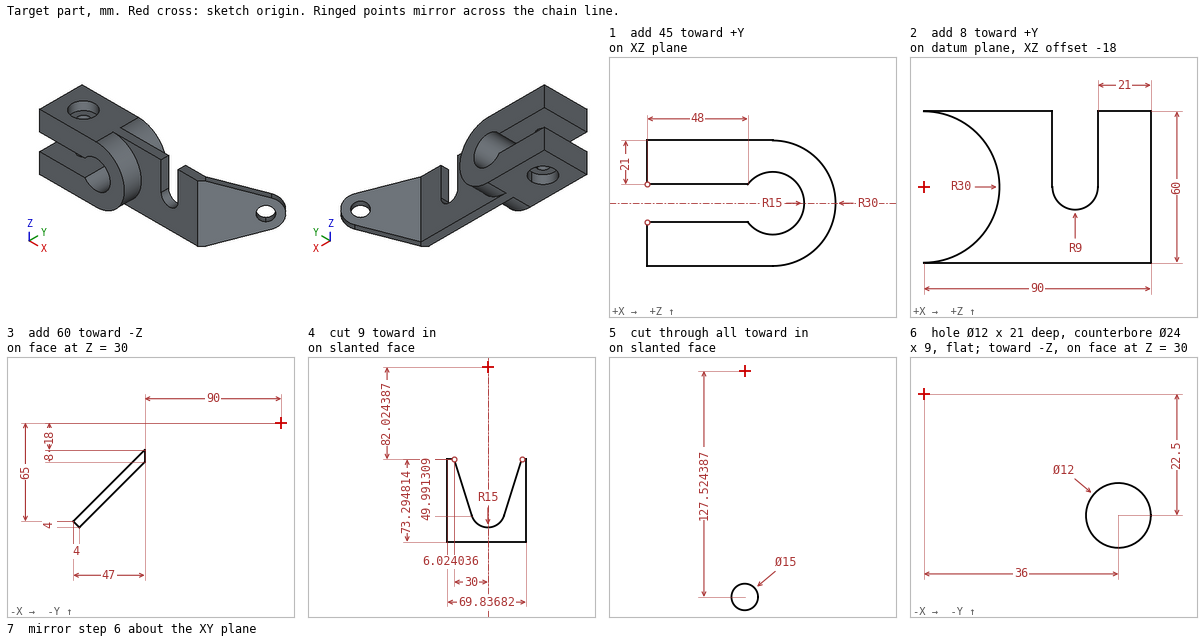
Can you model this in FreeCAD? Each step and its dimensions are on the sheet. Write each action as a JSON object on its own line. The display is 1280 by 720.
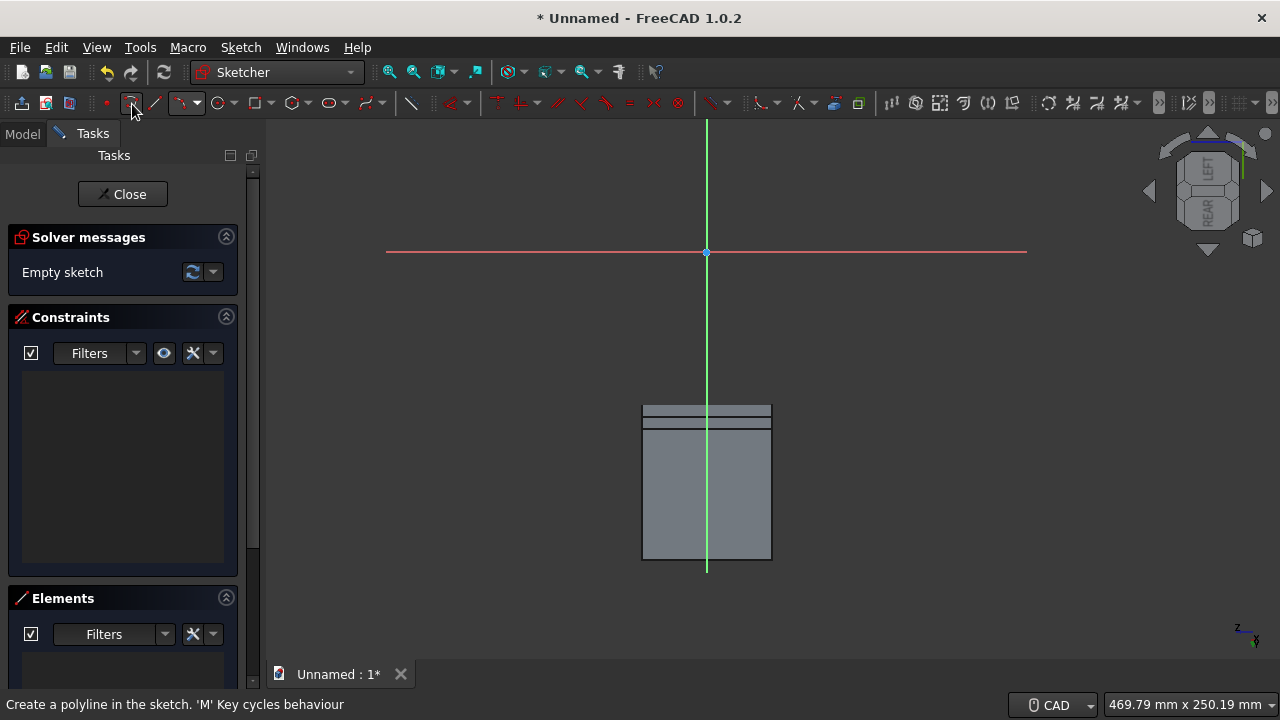
{"action": "left_click", "coordinate": [676, 537]}
{"action": "left_click", "coordinate": [642, 429]}
{"action": "left_click", "coordinate": [629, 429]}
{"action": "left_click", "coordinate": [629, 587]}
{"action": "left_click", "coordinate": [780, 587]}
{"action": "left_click", "coordinate": [780, 429]}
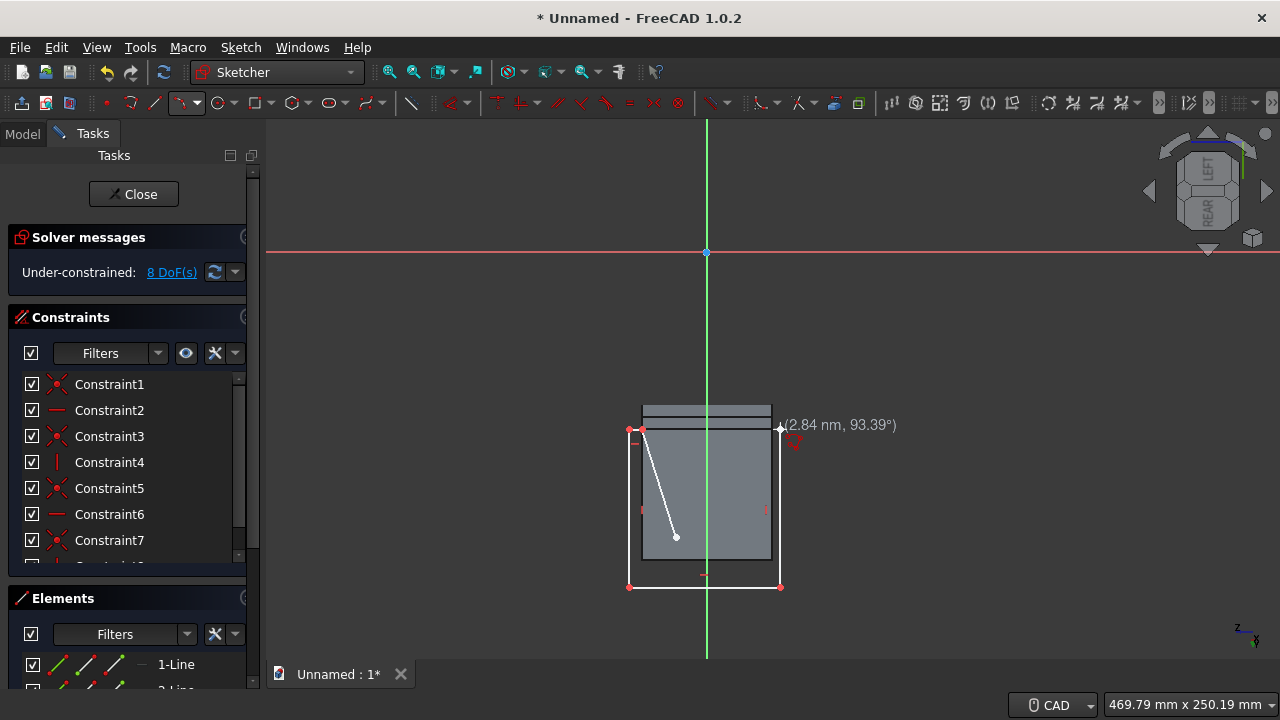
{"action": "scroll", "coordinate": [772, 429], "scroll_direction": "up", "scroll_amount": 4}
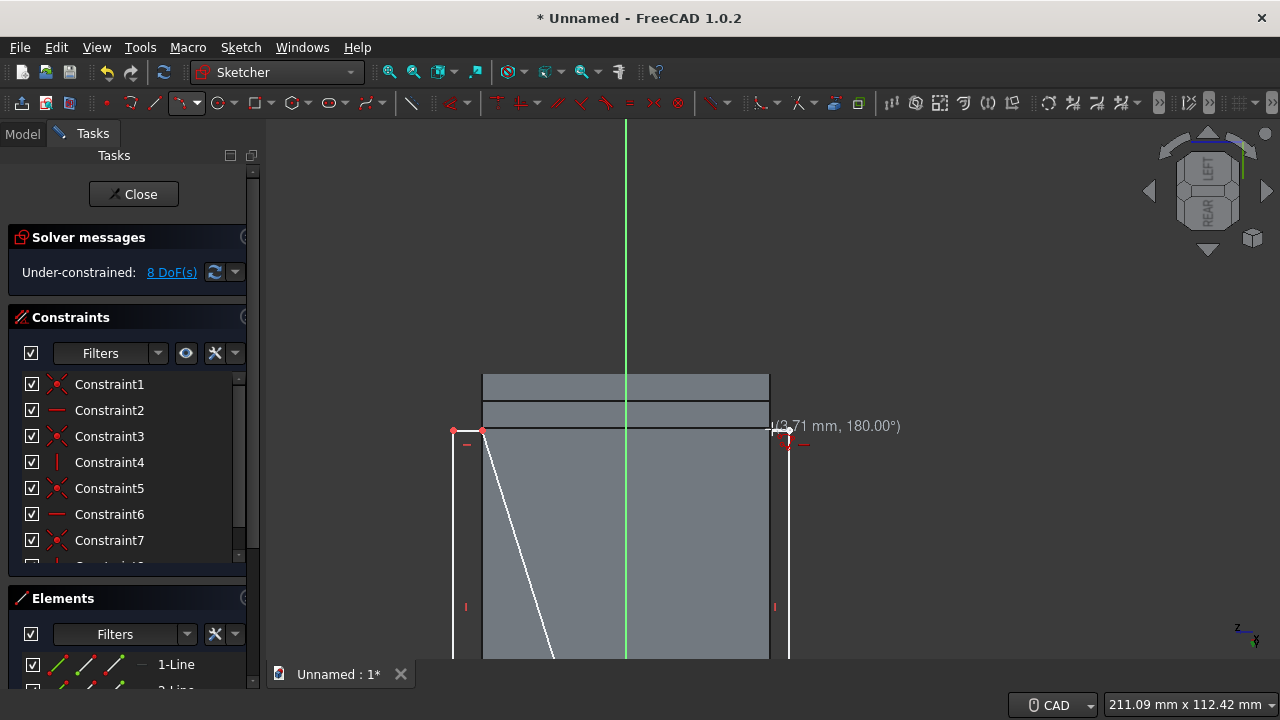
{"action": "left_click", "coordinate": [770, 428]}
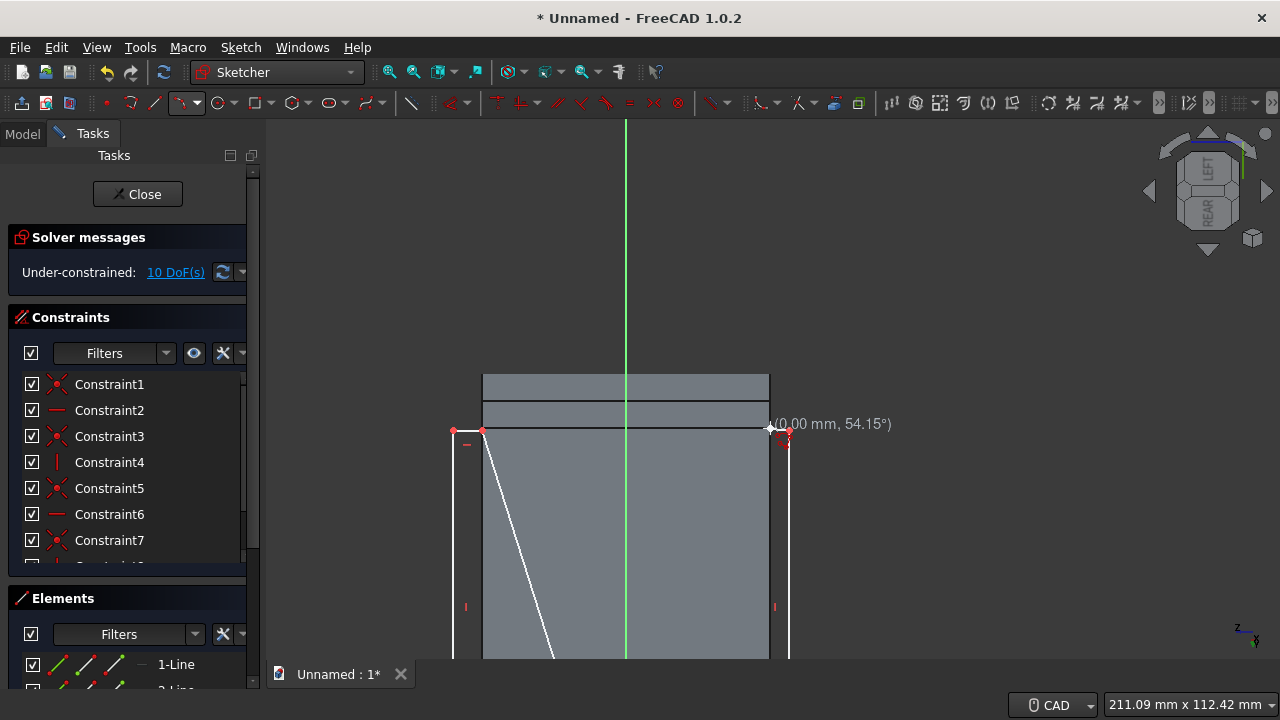
{"action": "scroll", "coordinate": [773, 374], "scroll_direction": "down", "scroll_amount": 4}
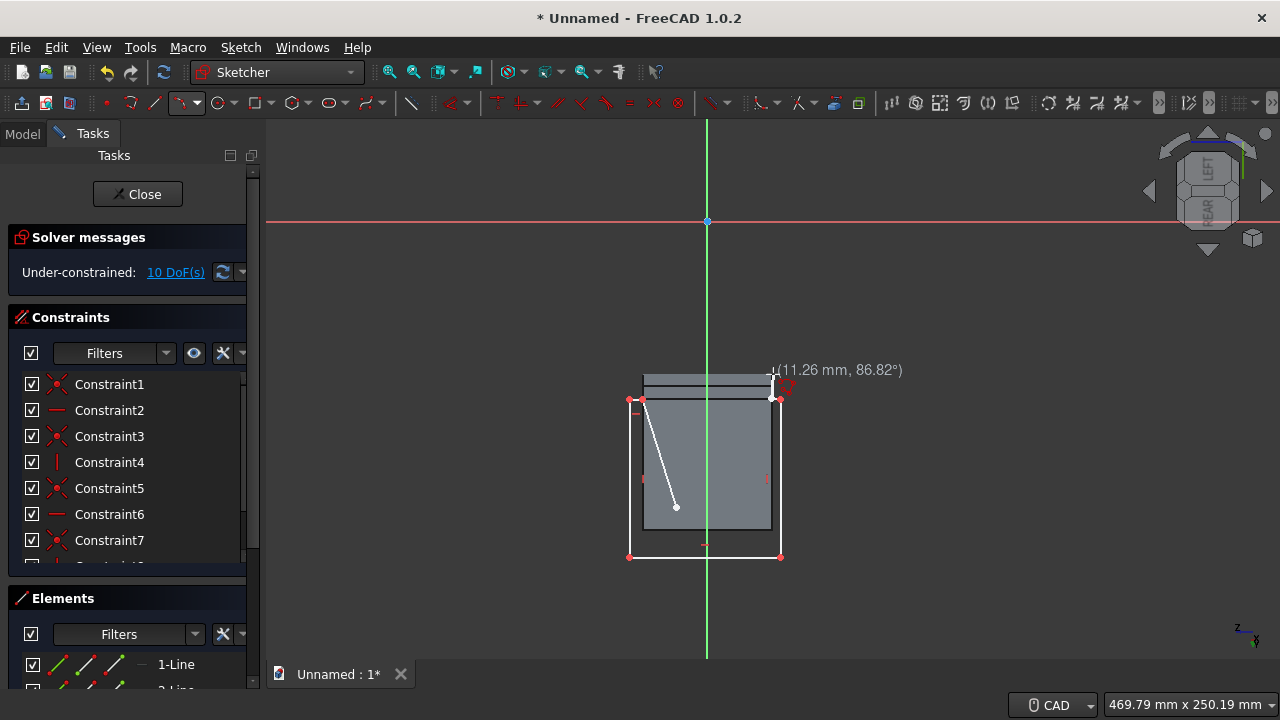
{"action": "left_click", "coordinate": [738, 507]}
{"action": "right_click", "coordinate": [738, 507]}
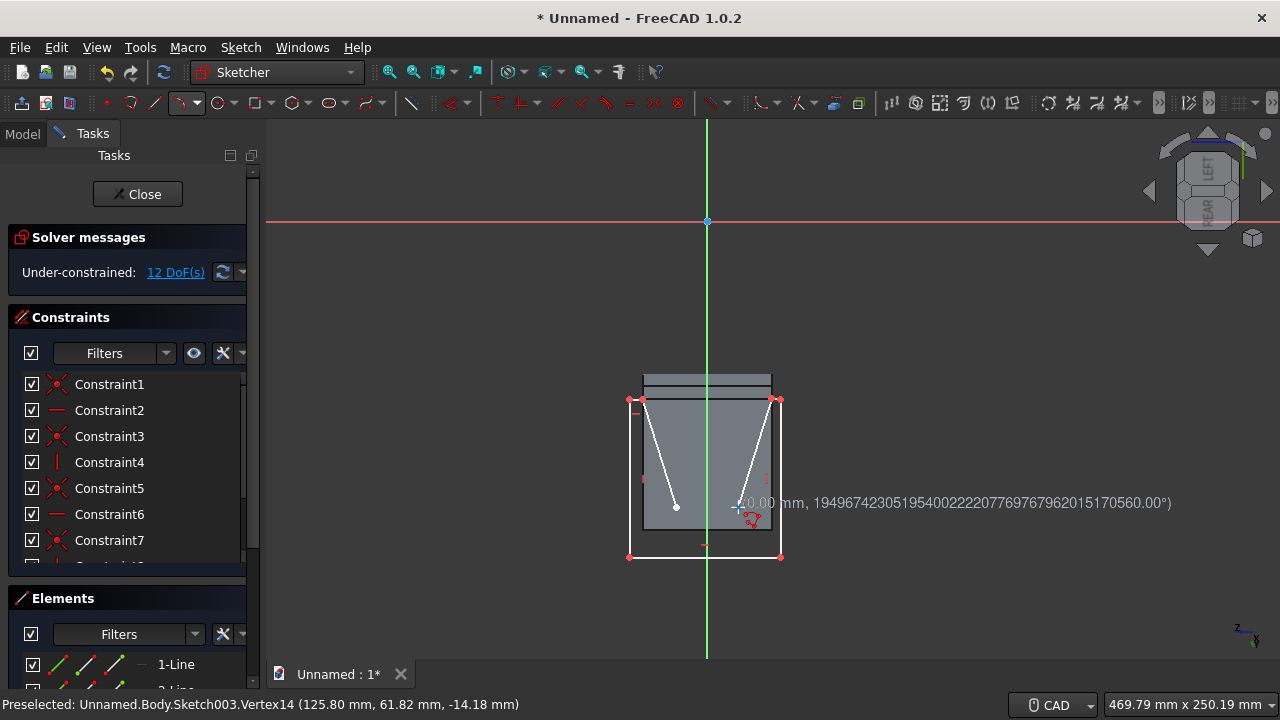
{"action": "left_click", "coordinate": [180, 104]}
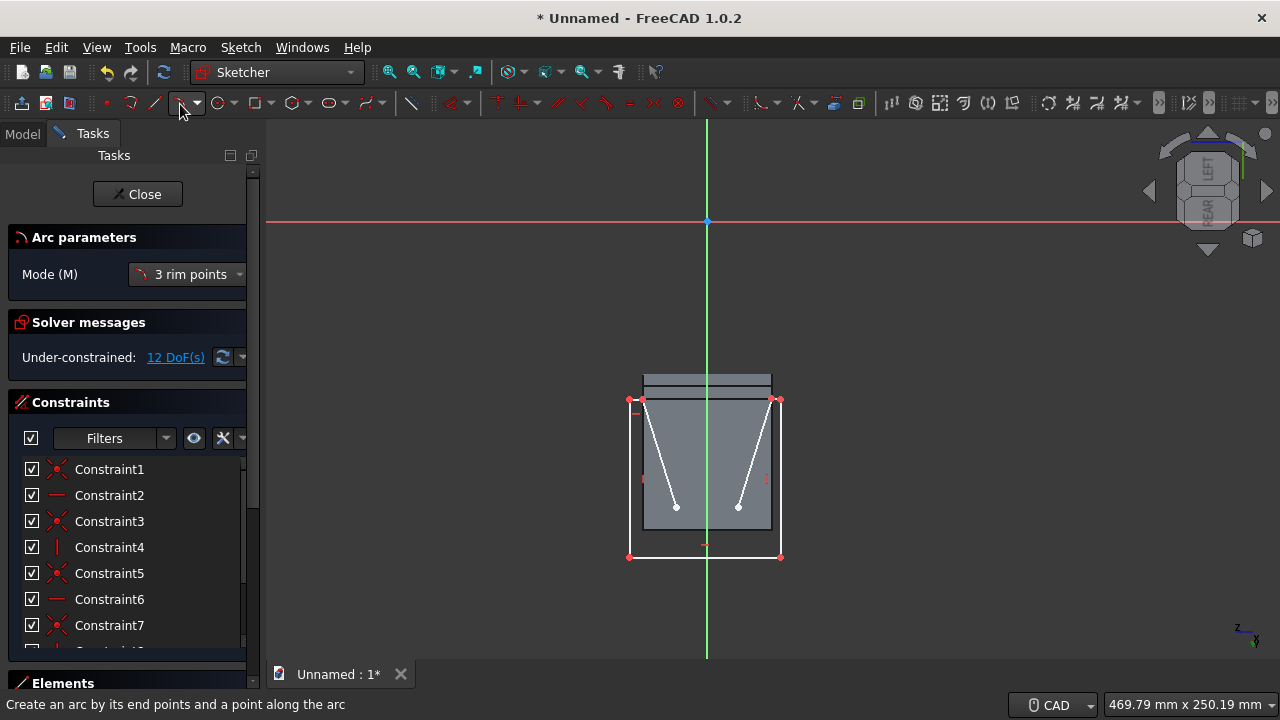
{"action": "left_click", "coordinate": [738, 508]}
{"action": "left_click", "coordinate": [677, 508]}
{"action": "left_click", "coordinate": [692, 525]}
{"action": "key", "text": "Escape"}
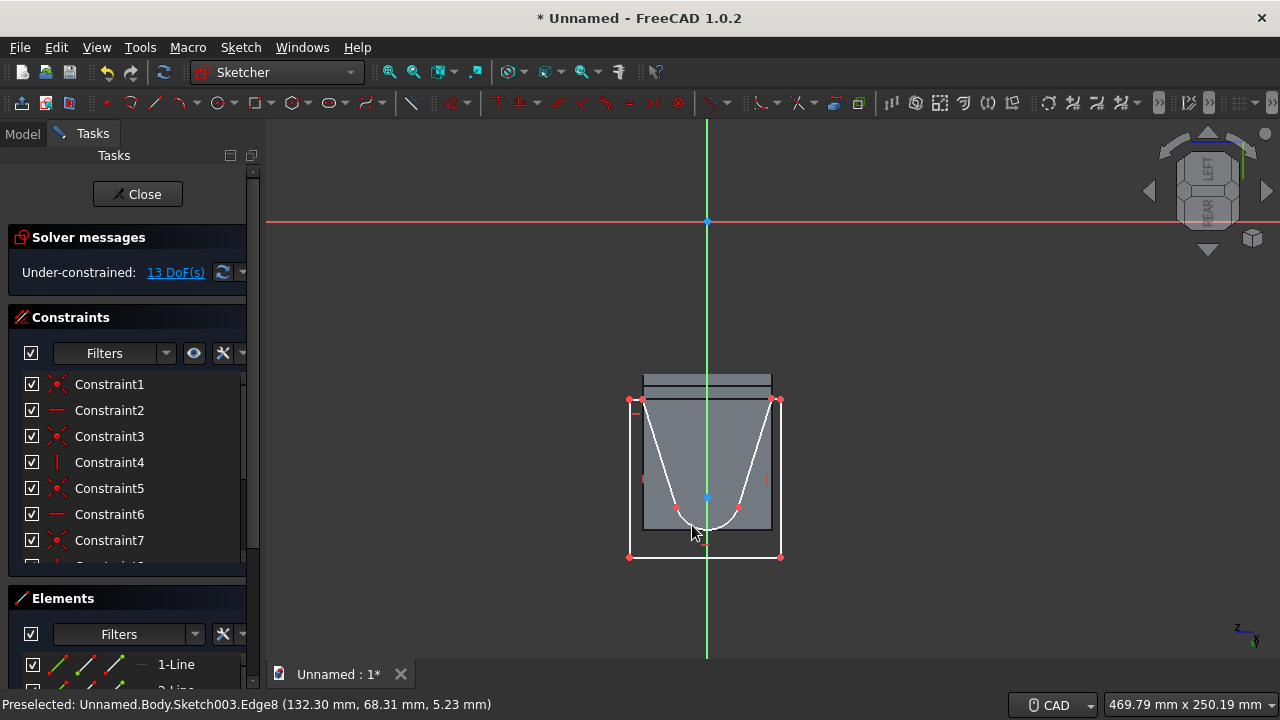
{"action": "left_click", "coordinate": [666, 475]}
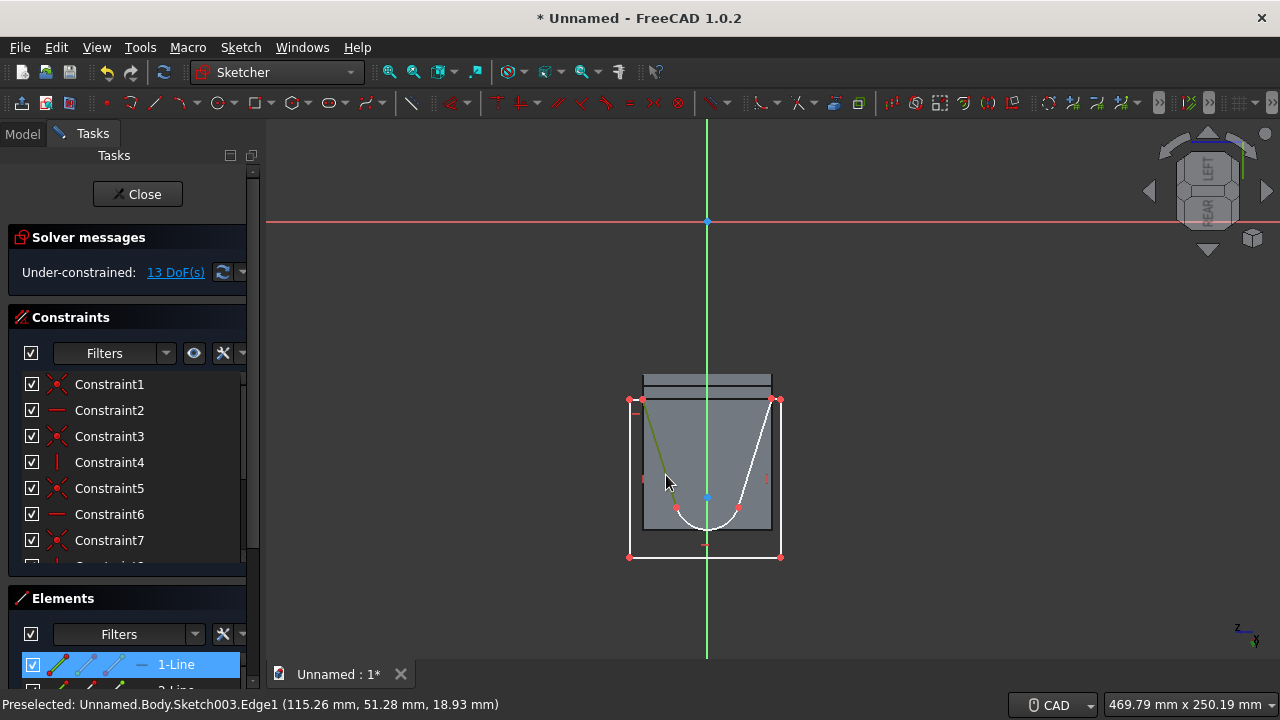
{"action": "left_click", "coordinate": [692, 526]}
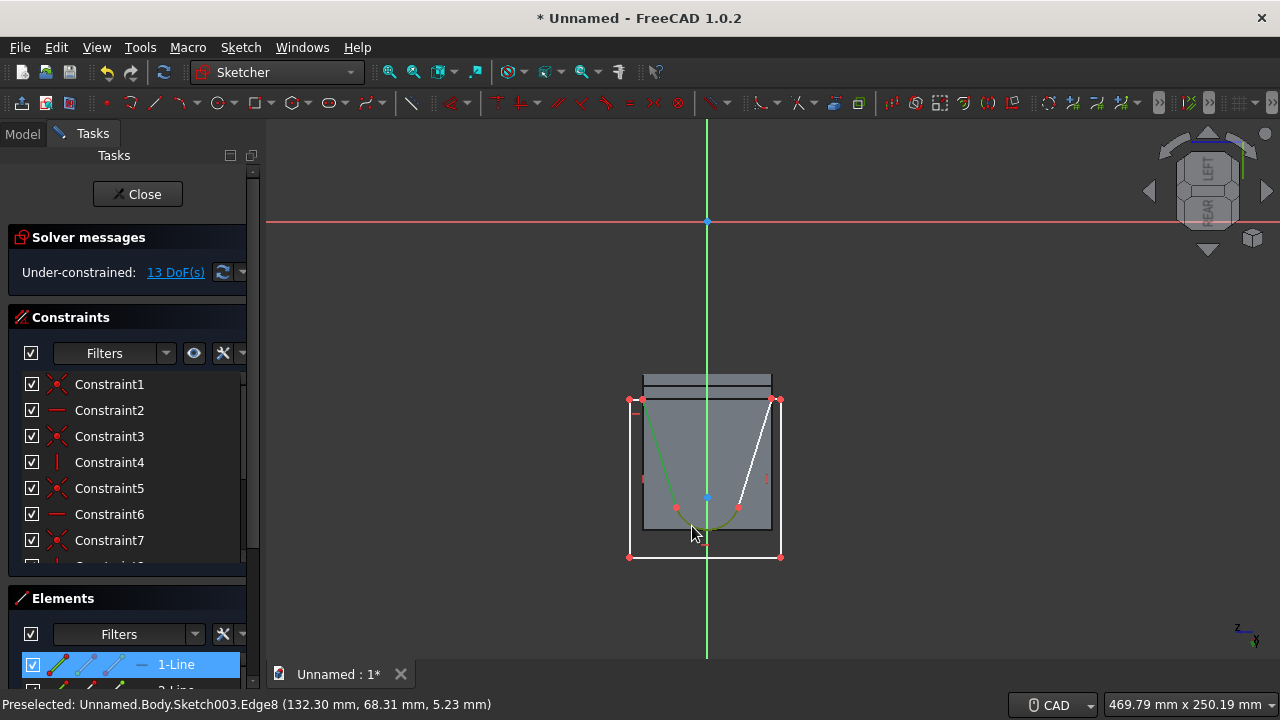
{"action": "left_click", "coordinate": [606, 104]}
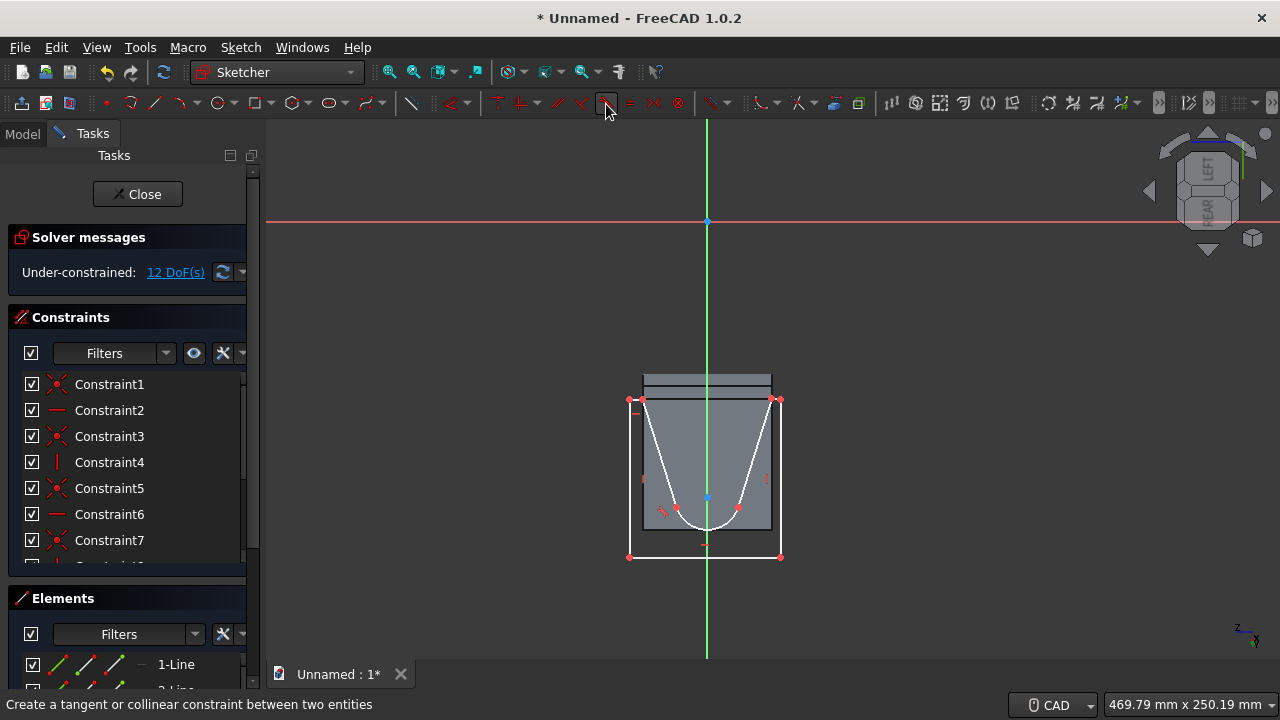
{"action": "left_click", "coordinate": [762, 432]}